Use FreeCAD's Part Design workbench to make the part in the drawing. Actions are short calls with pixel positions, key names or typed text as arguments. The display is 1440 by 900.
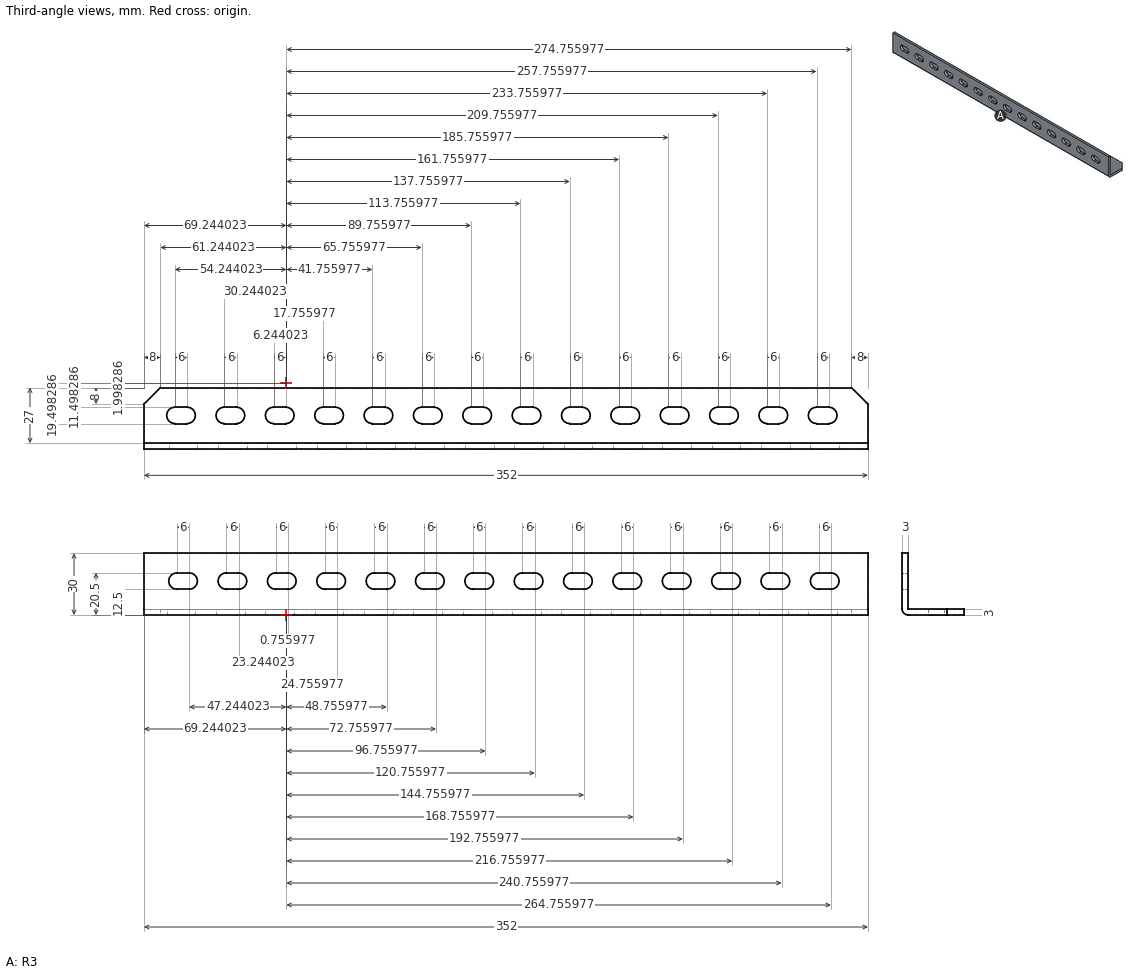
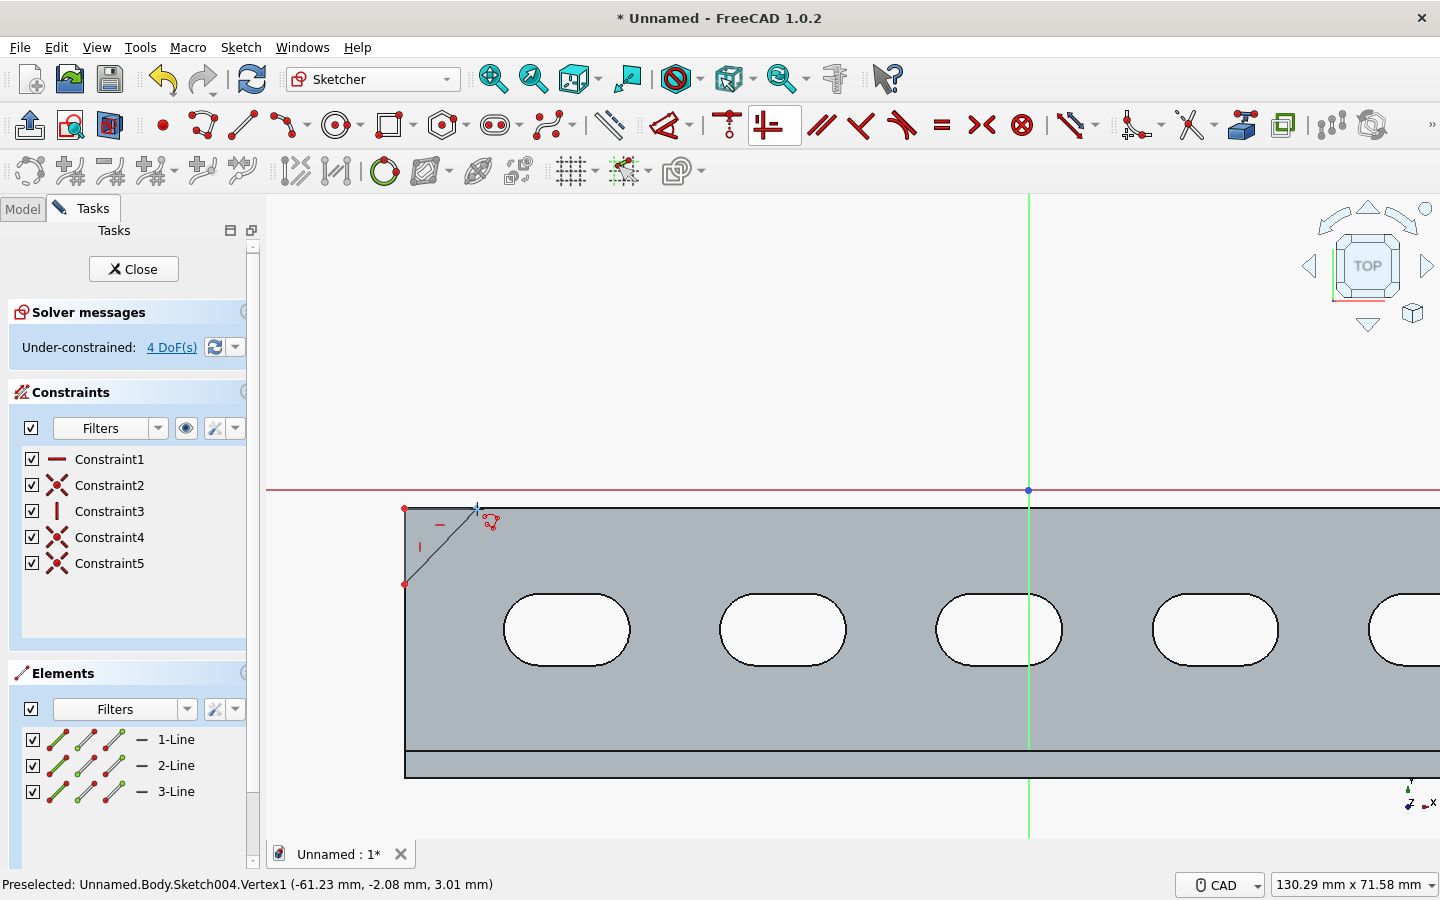
scroll(479, 512, down, 8)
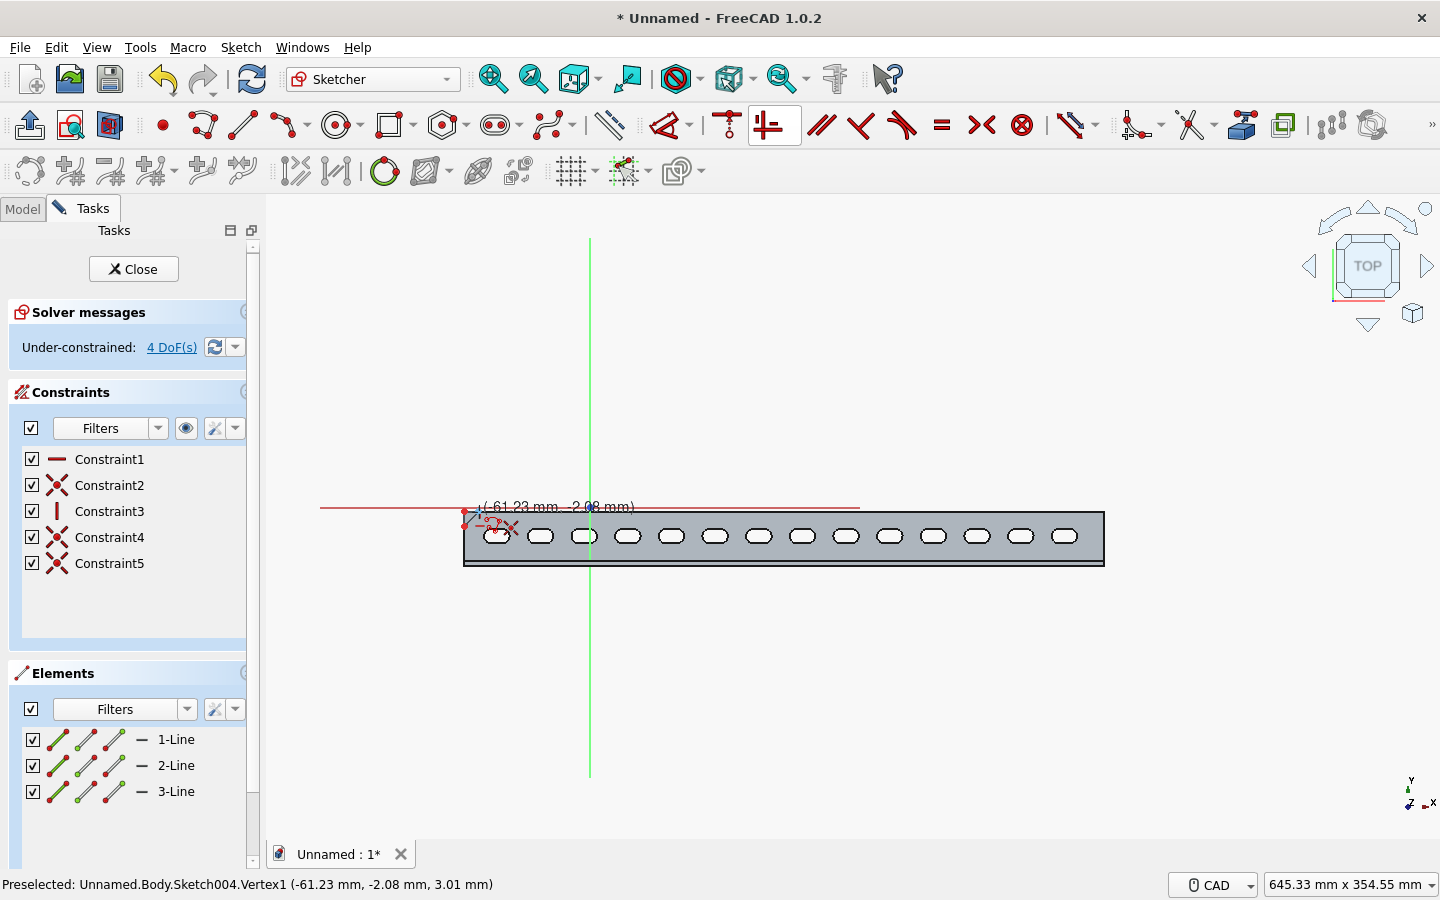
scroll(1090, 512, up, 8)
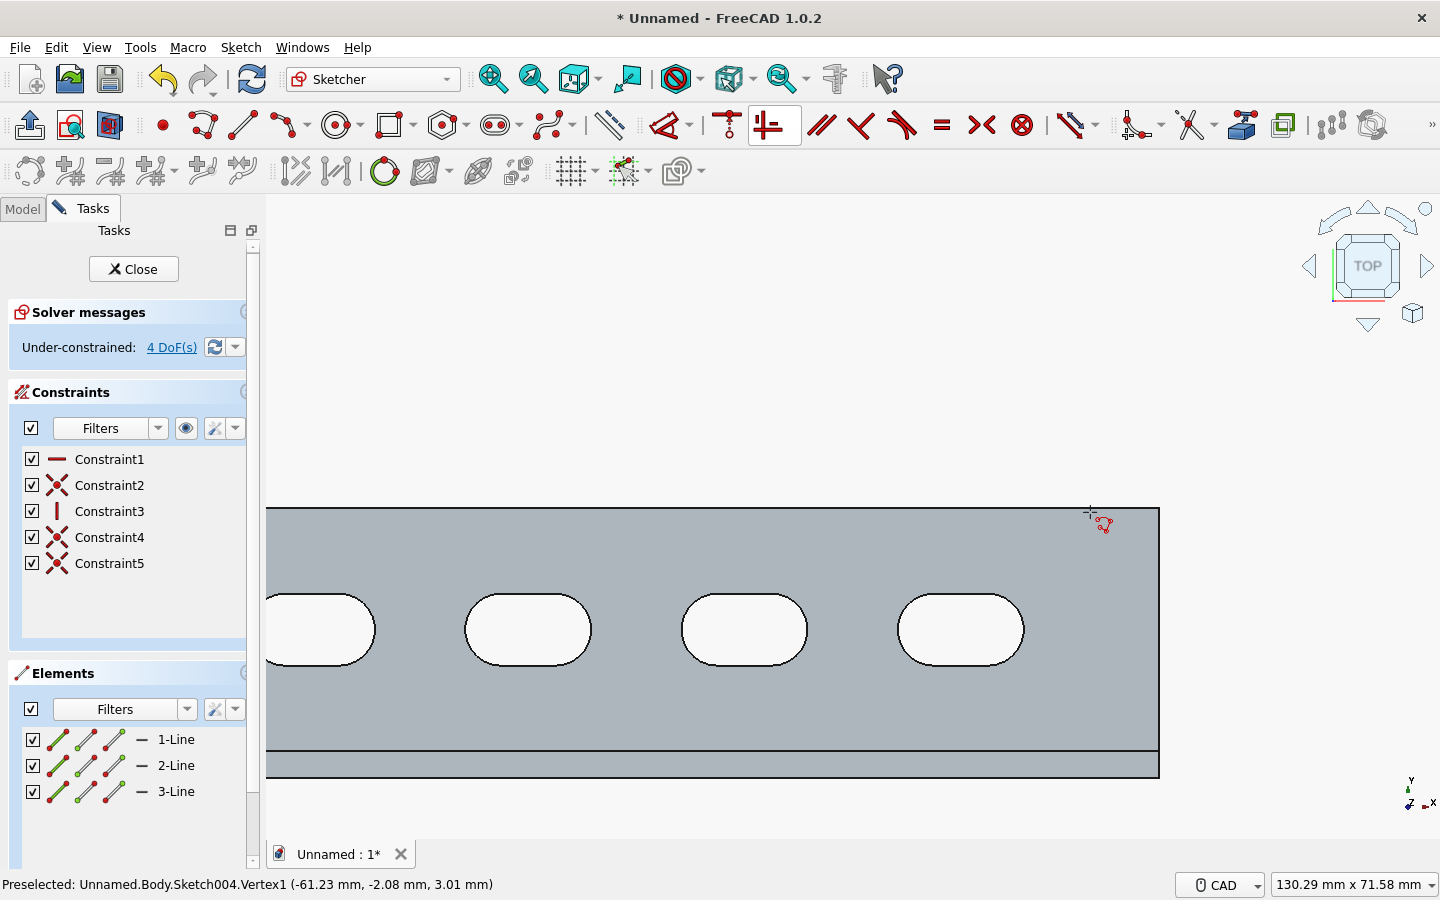
click(1087, 508)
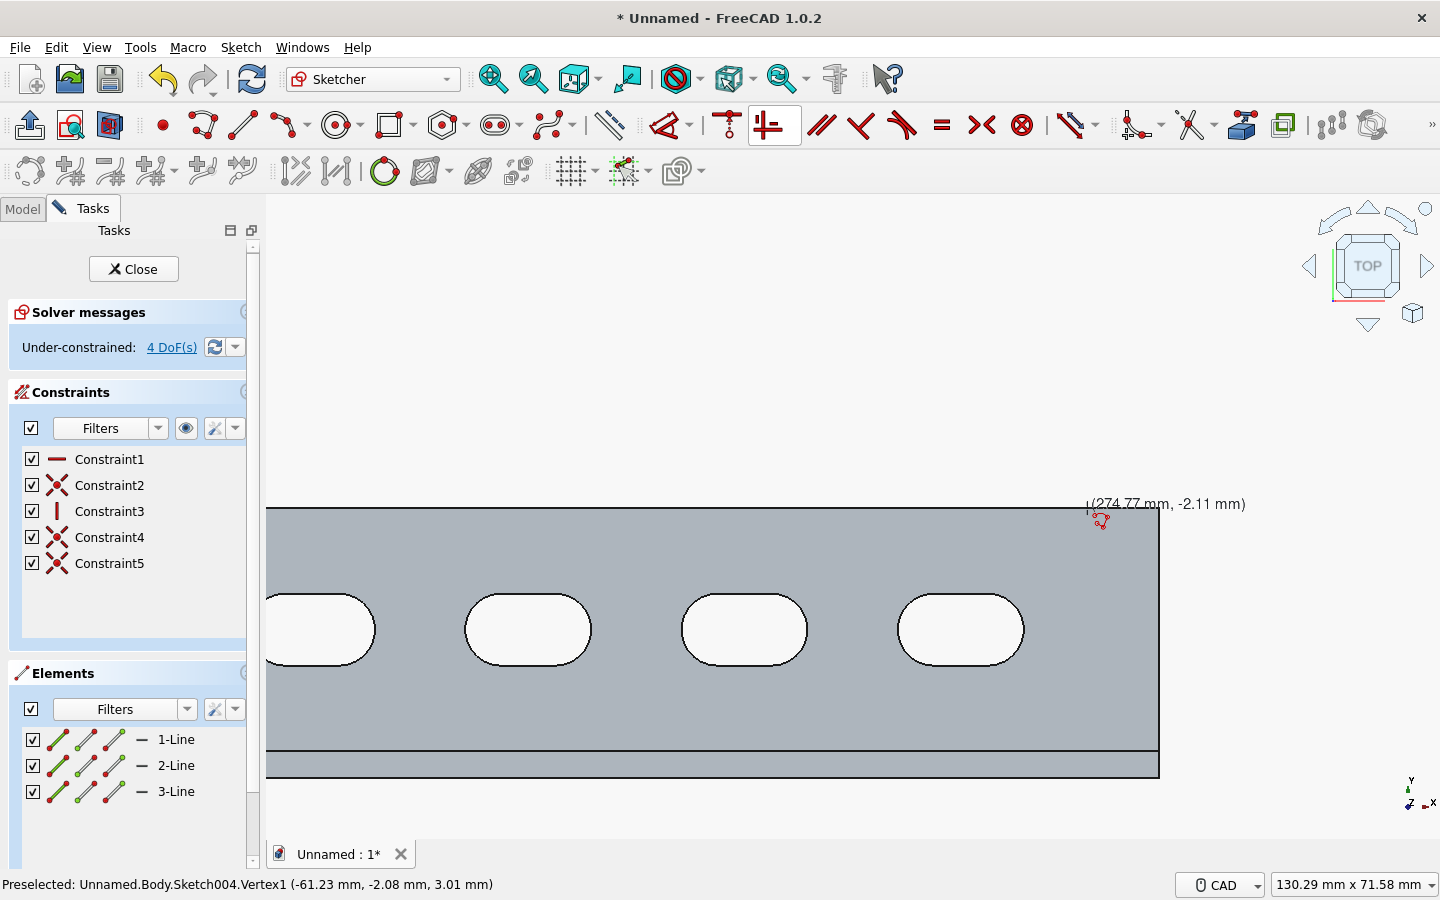
scroll(1091, 512, down, 8)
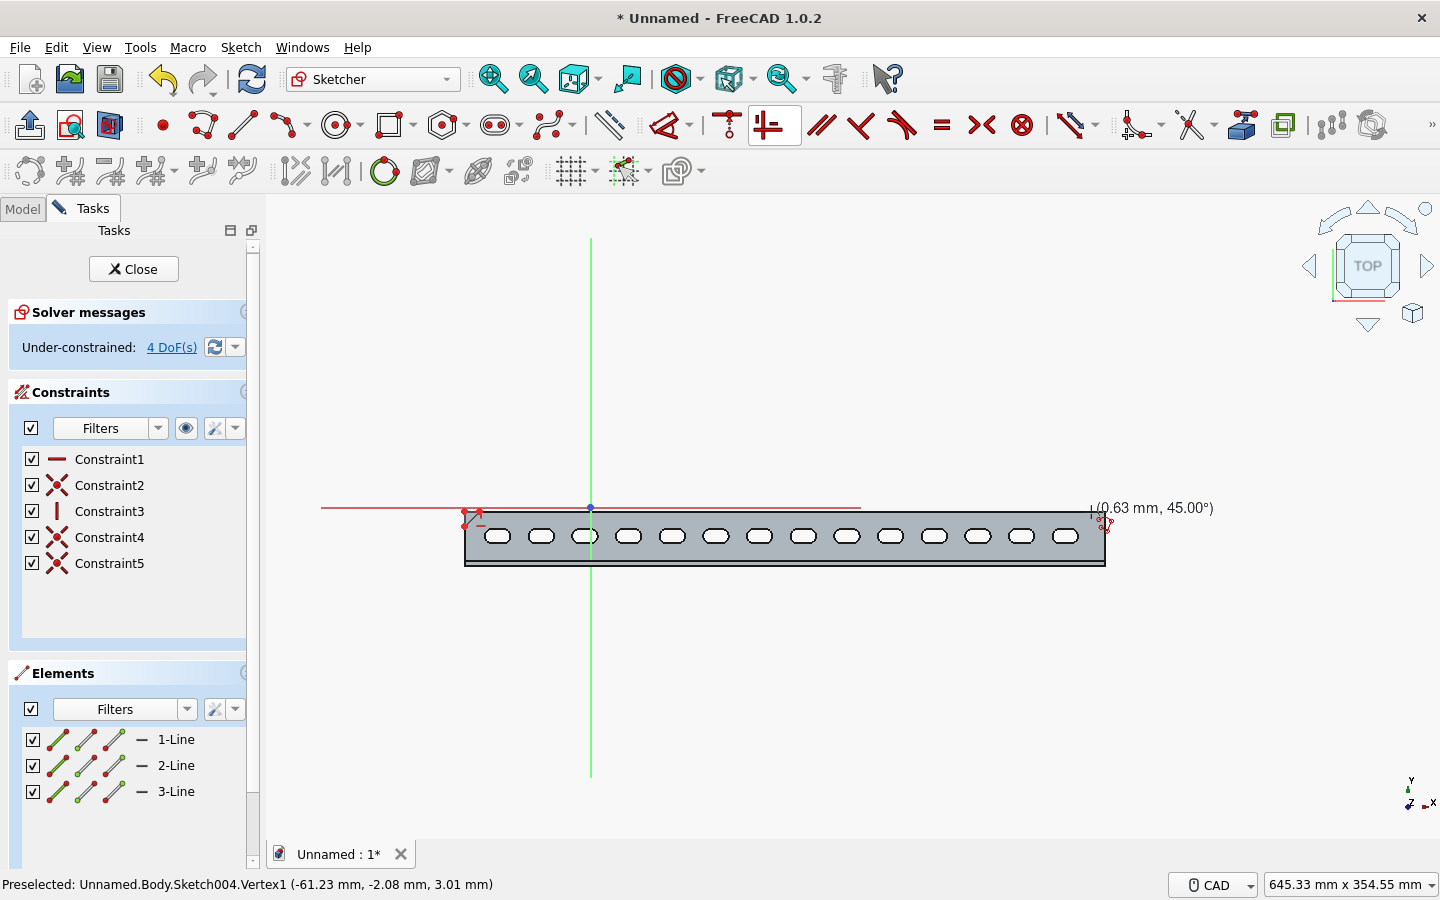
click(1105, 526)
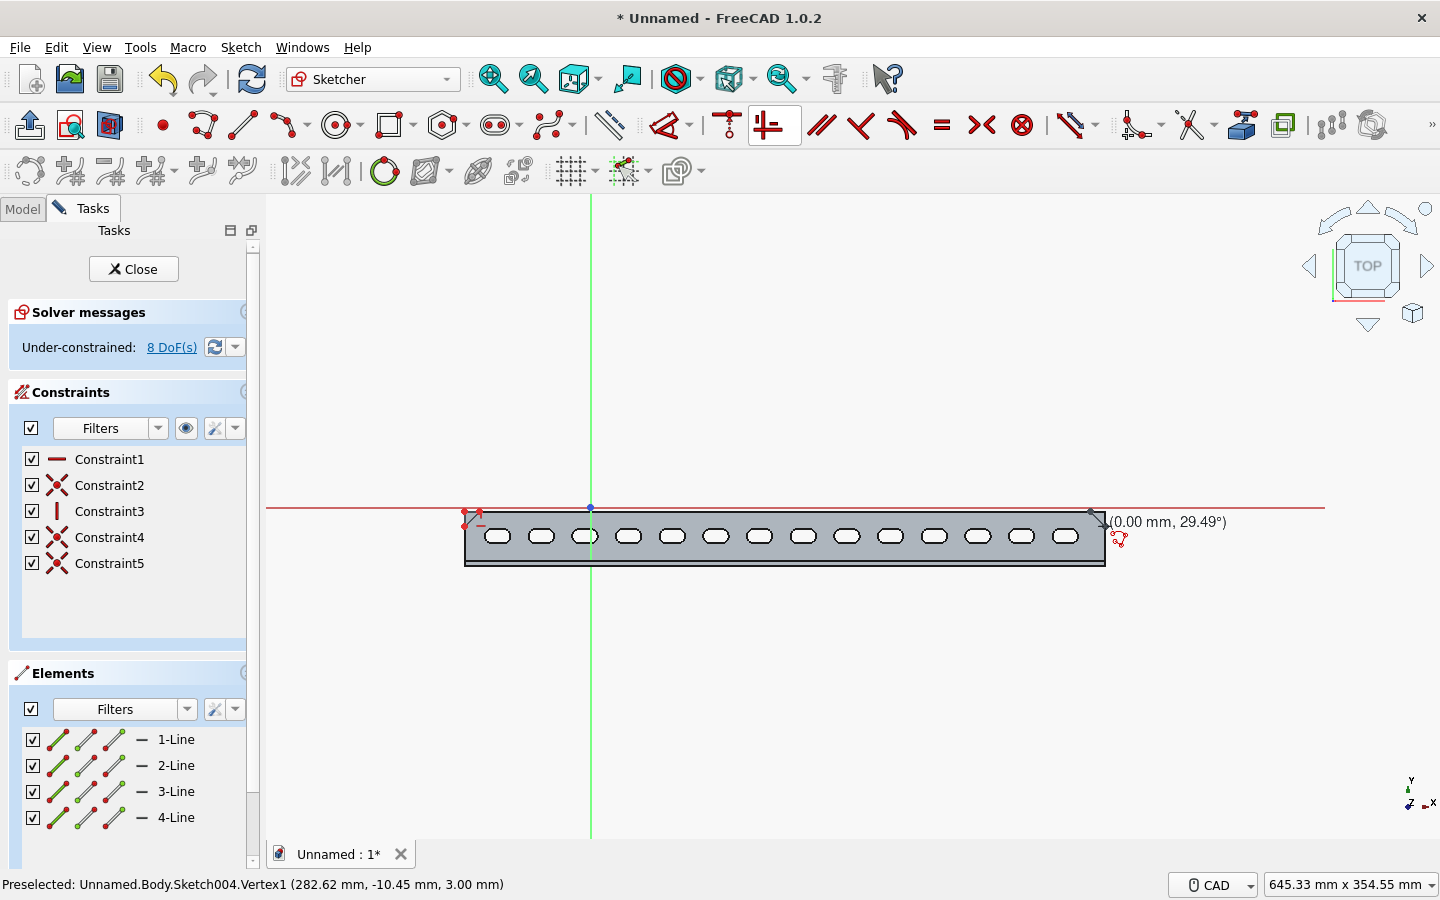
scroll(1105, 512, up, 8)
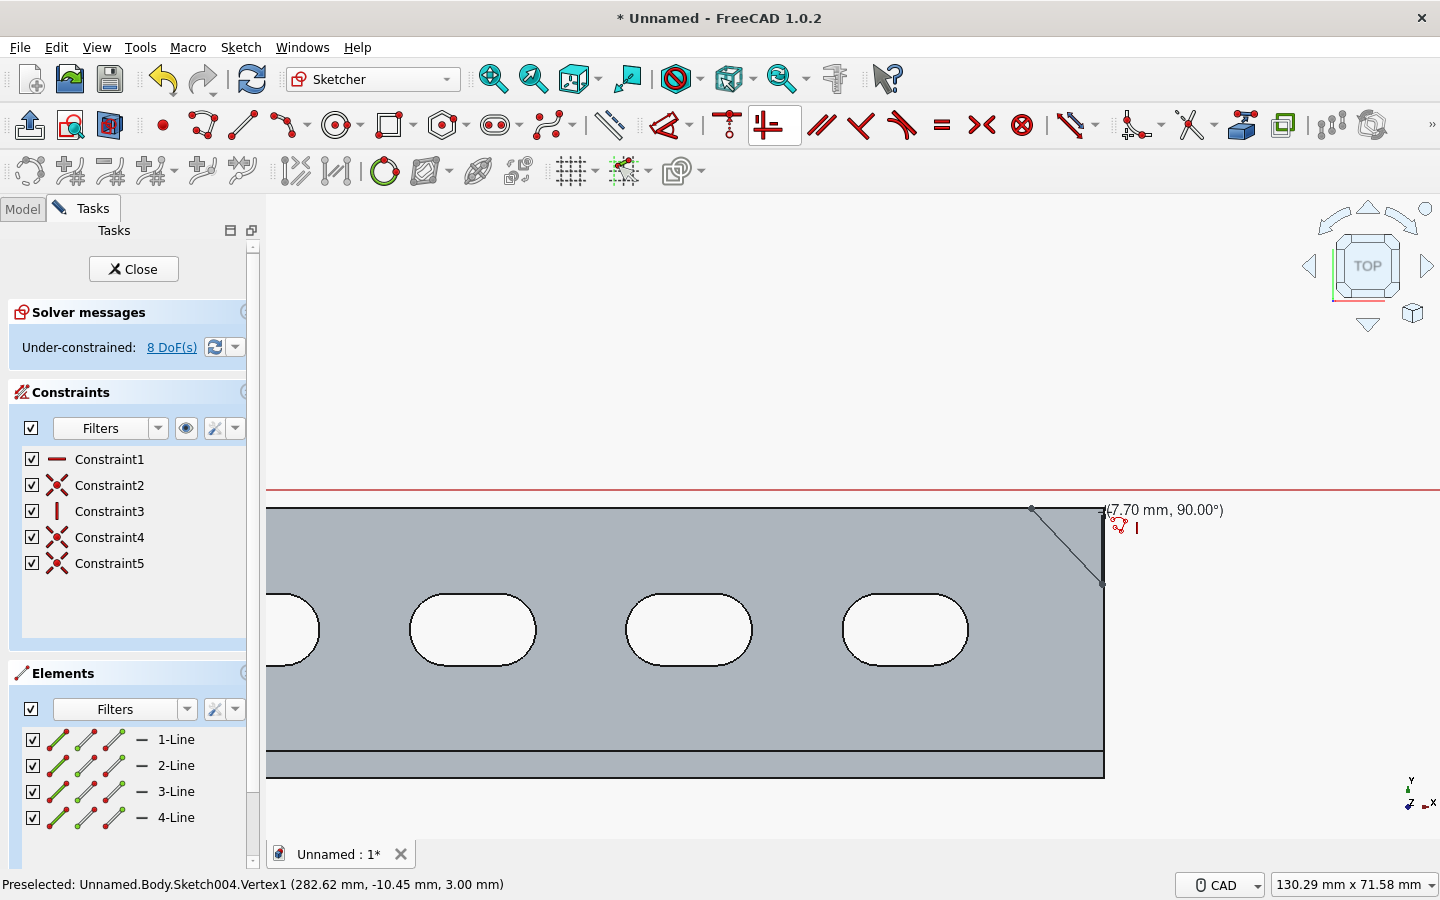
click(1102, 508)
click(1032, 509)
key(Escape)
key(Escape)